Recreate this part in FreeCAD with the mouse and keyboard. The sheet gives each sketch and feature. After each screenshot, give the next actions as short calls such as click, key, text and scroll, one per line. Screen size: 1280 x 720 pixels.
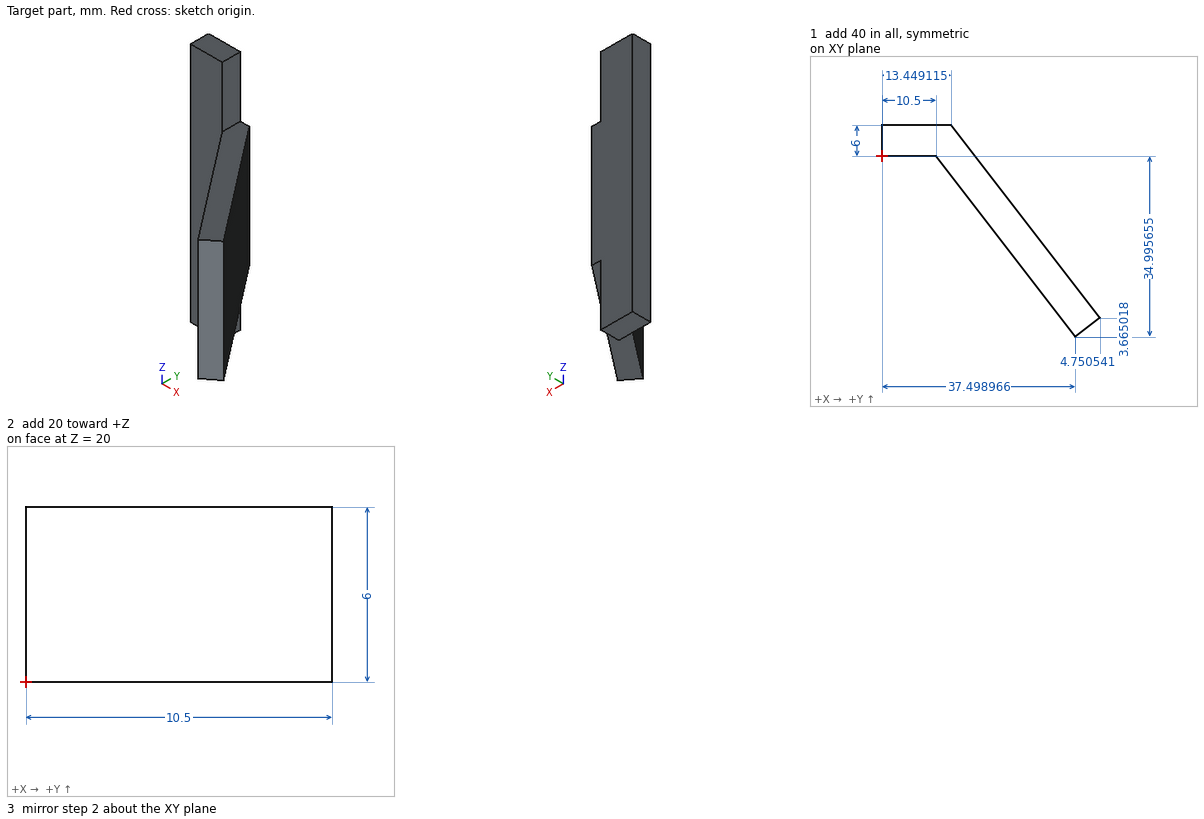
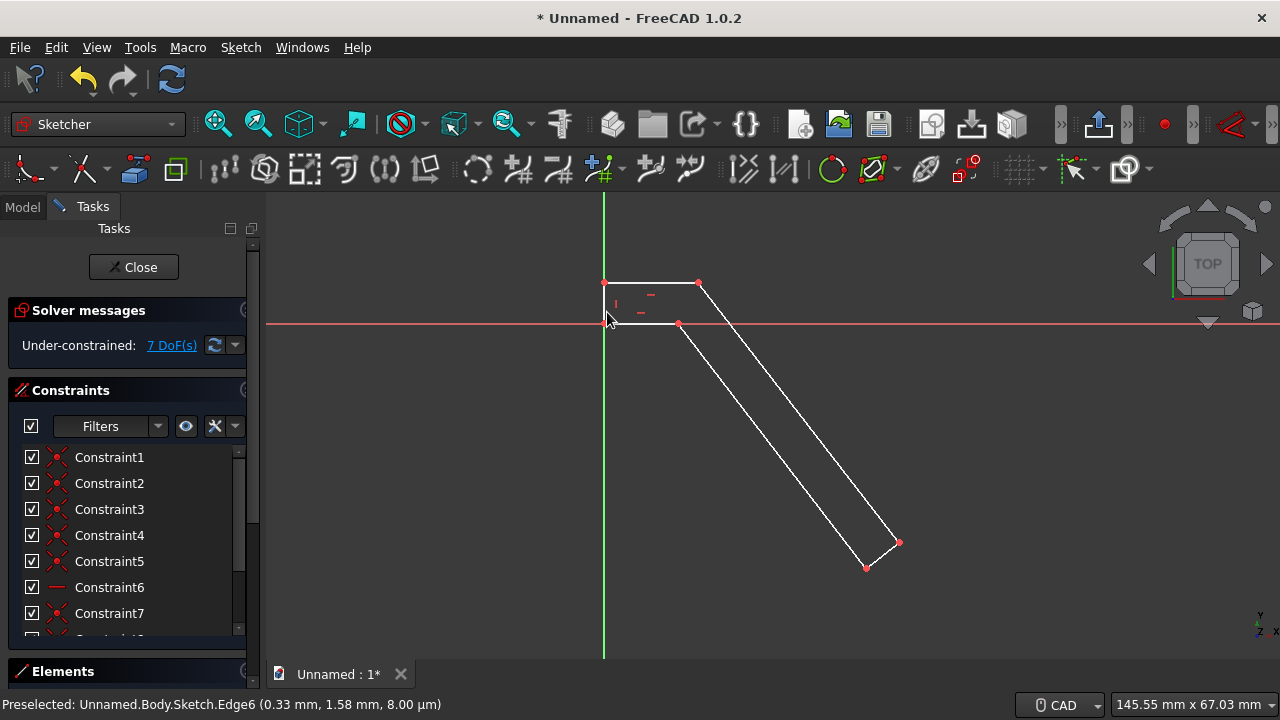
click(1232, 124)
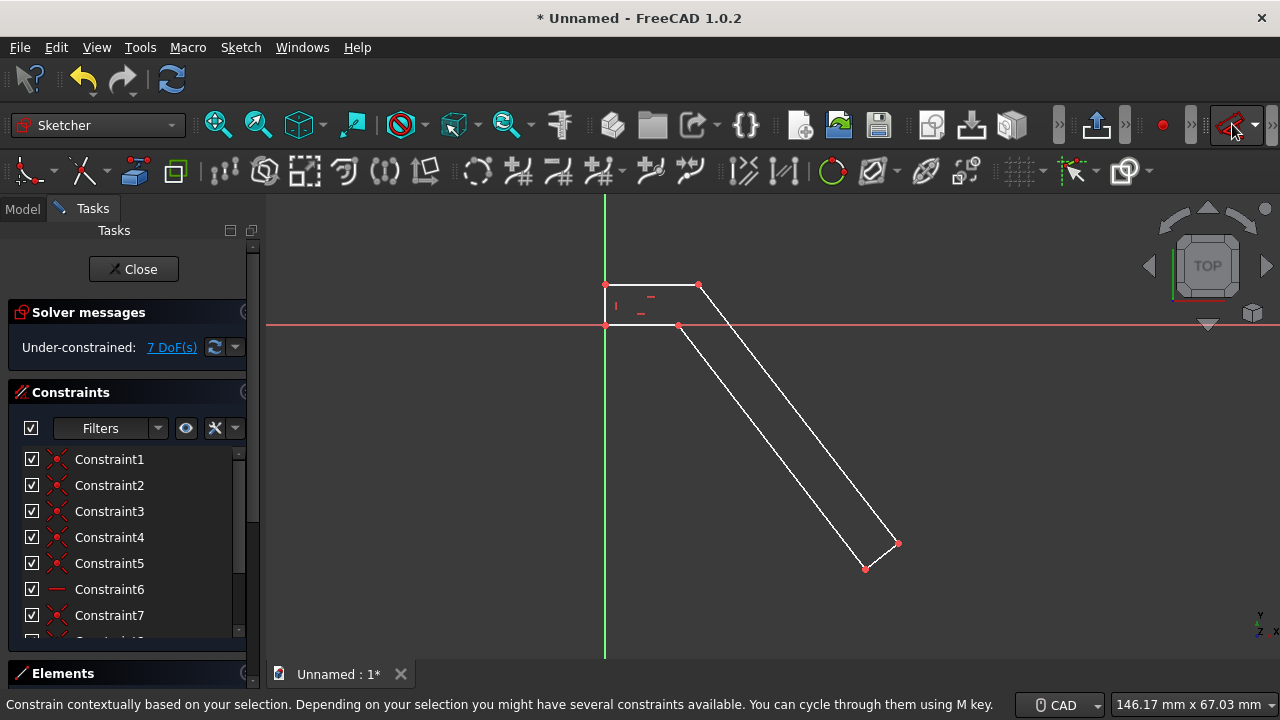
click(605, 297)
click(571, 305)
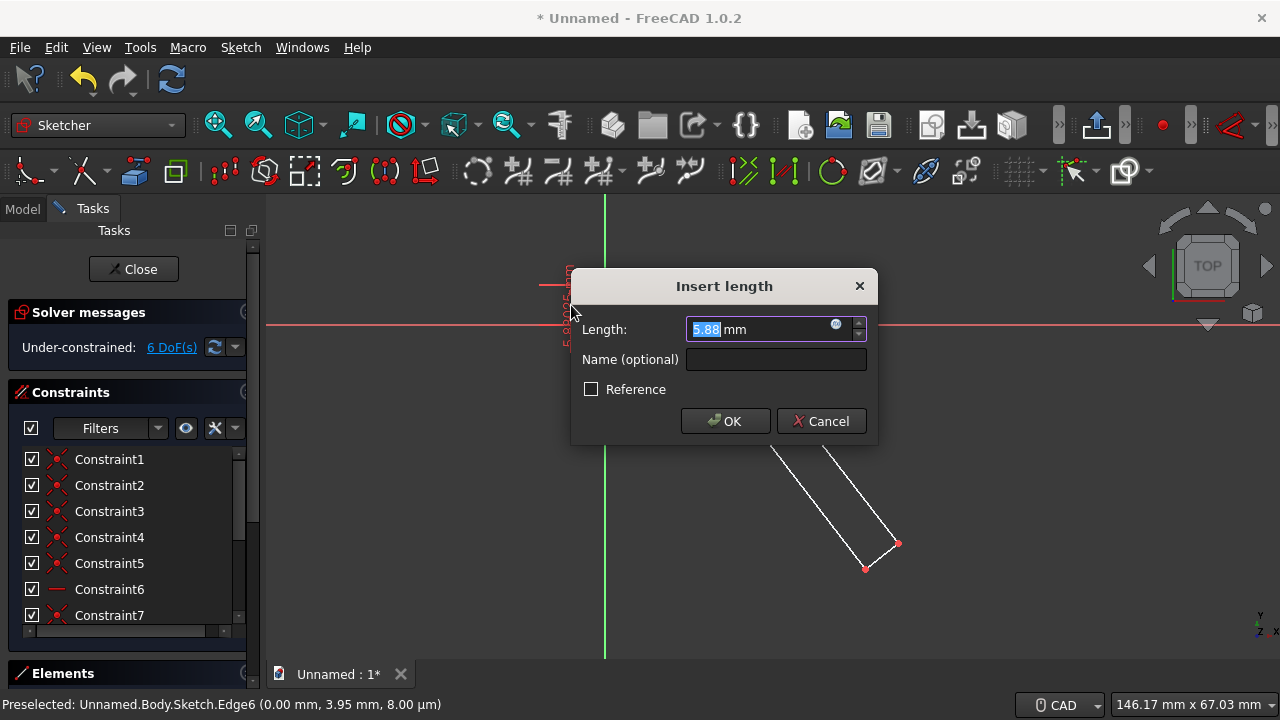
text(6)
key(Return)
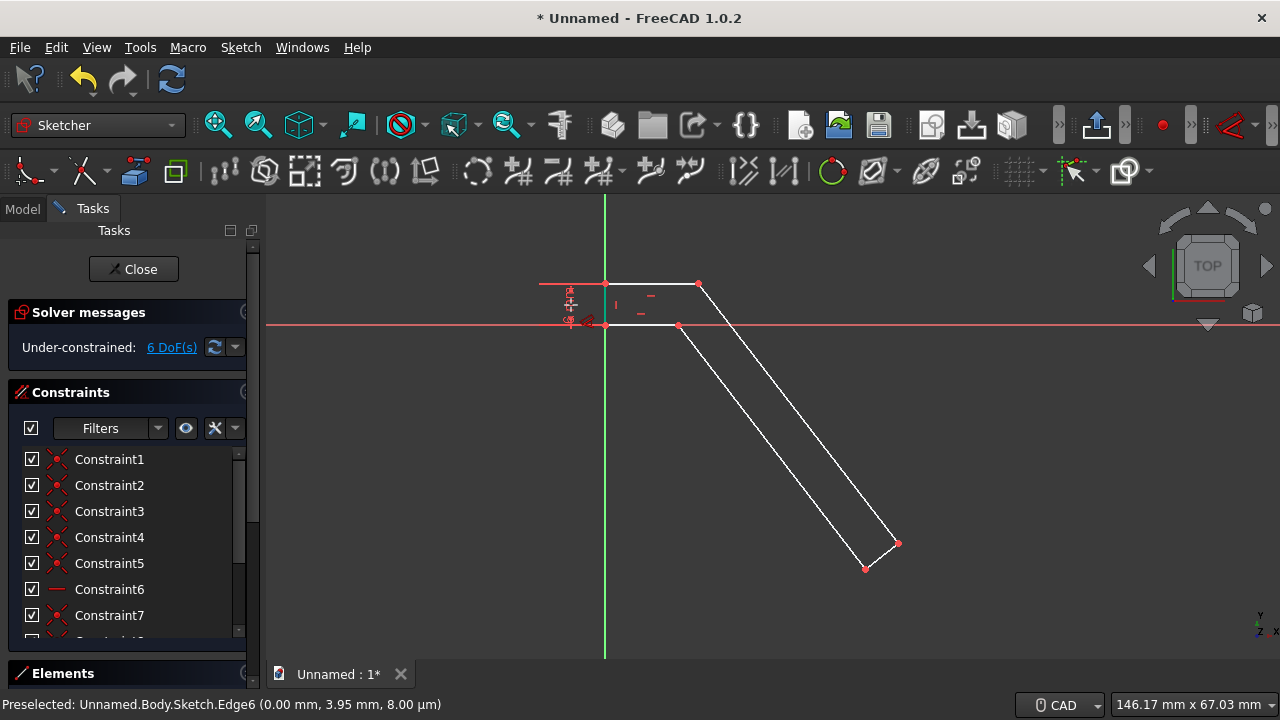
click(627, 325)
click(642, 359)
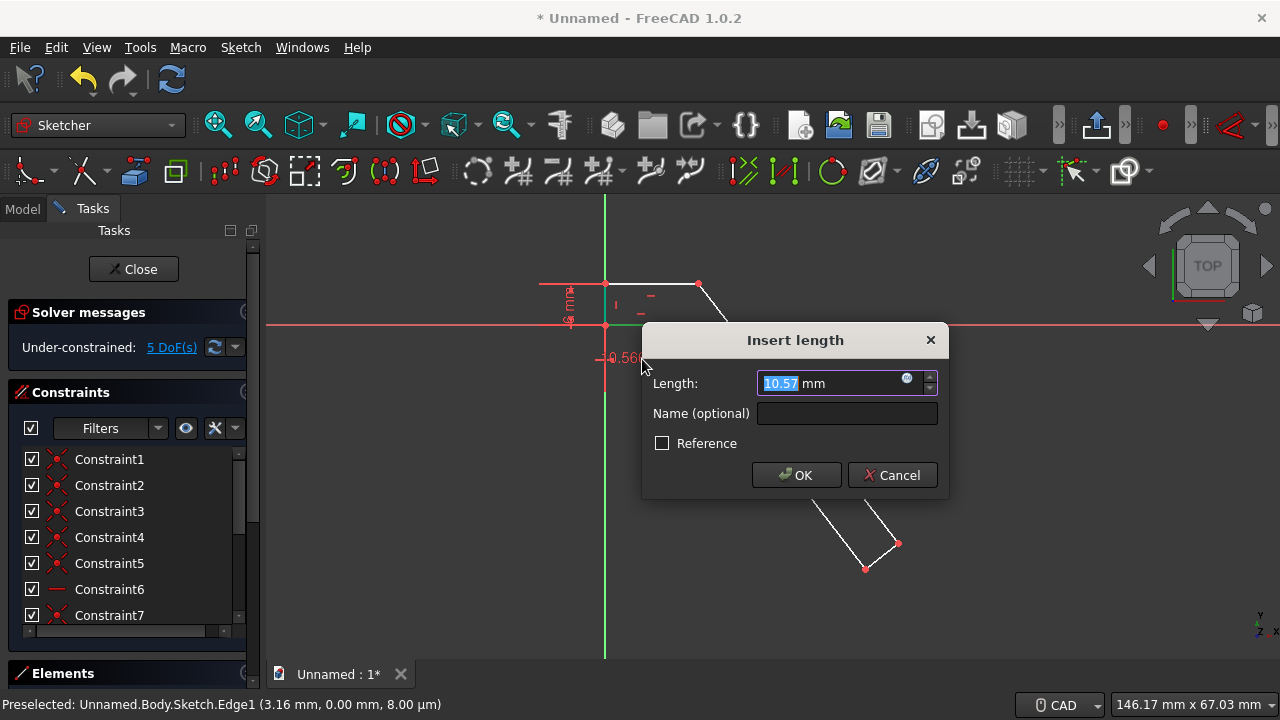
text(10.5)
key(Return)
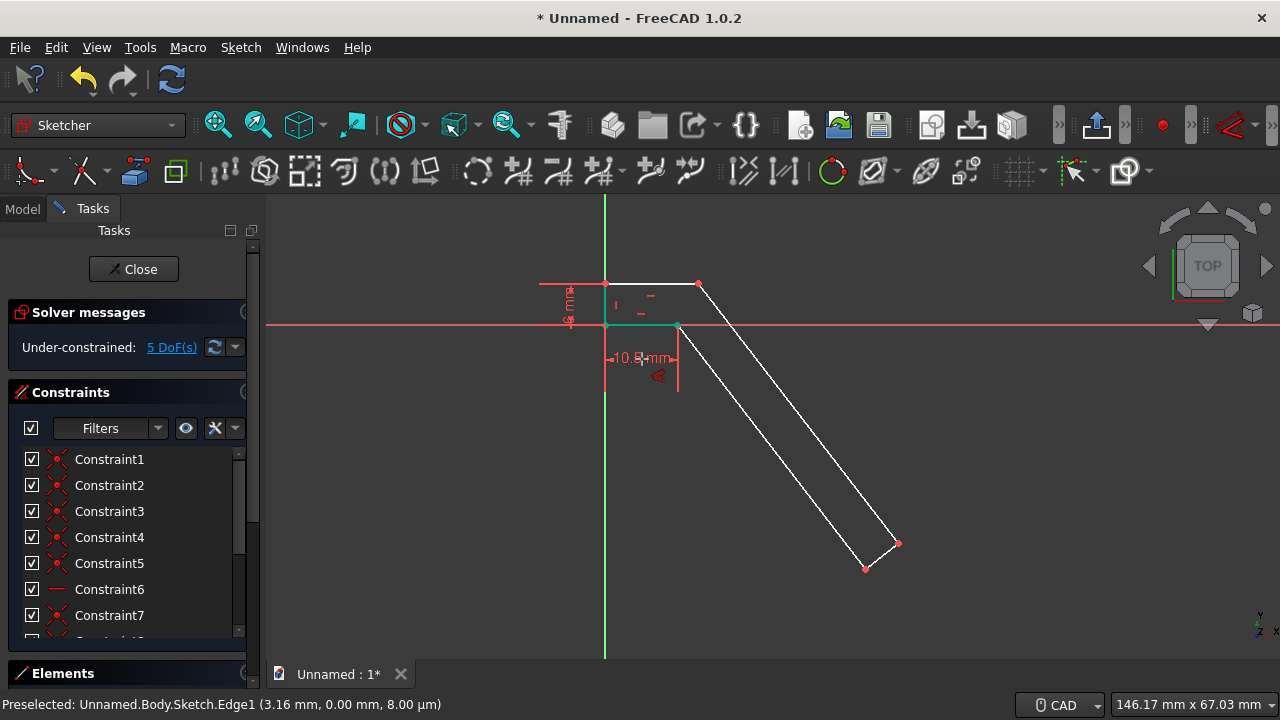
click(670, 284)
click(652, 250)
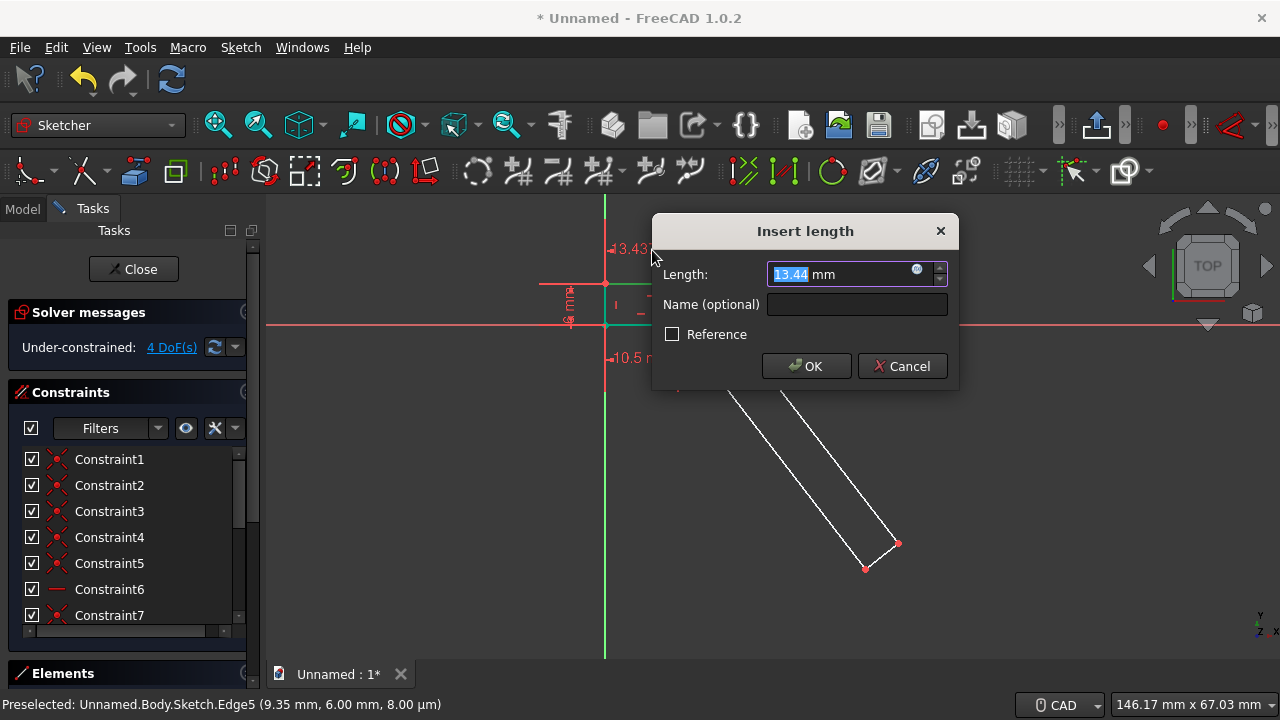
text(13.449115)
key(Return)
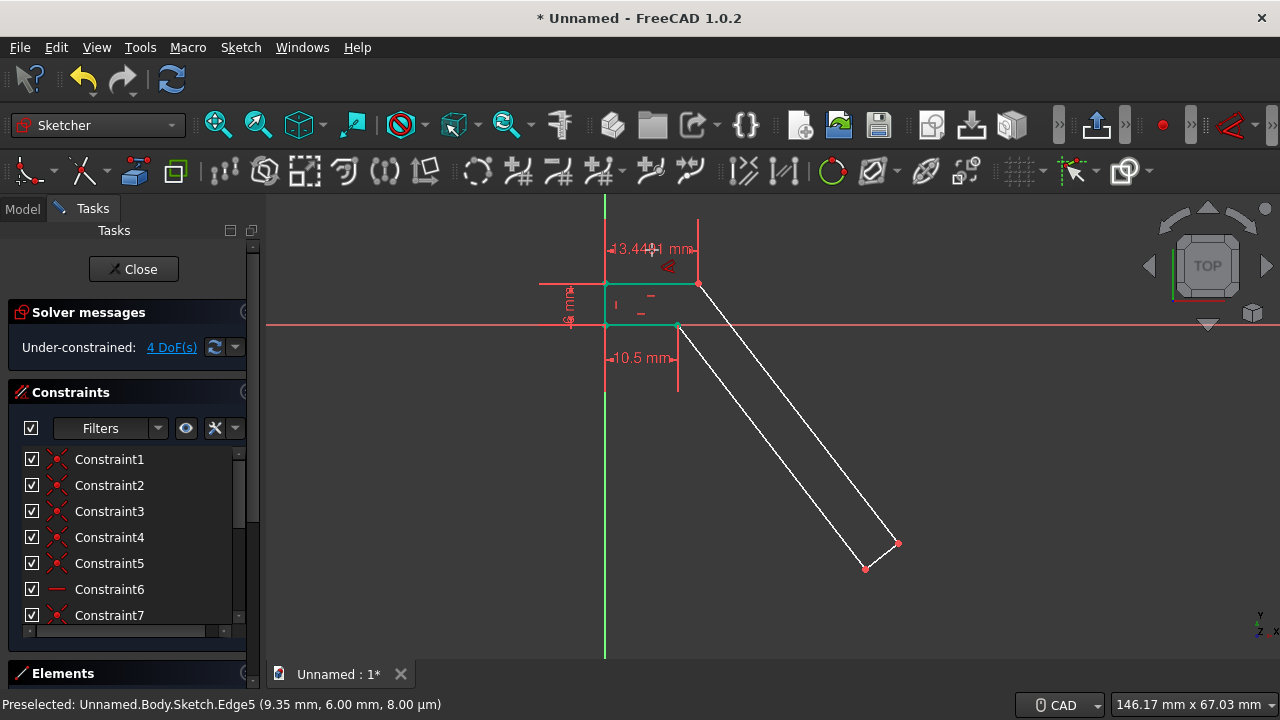
click(875, 562)
click(882, 603)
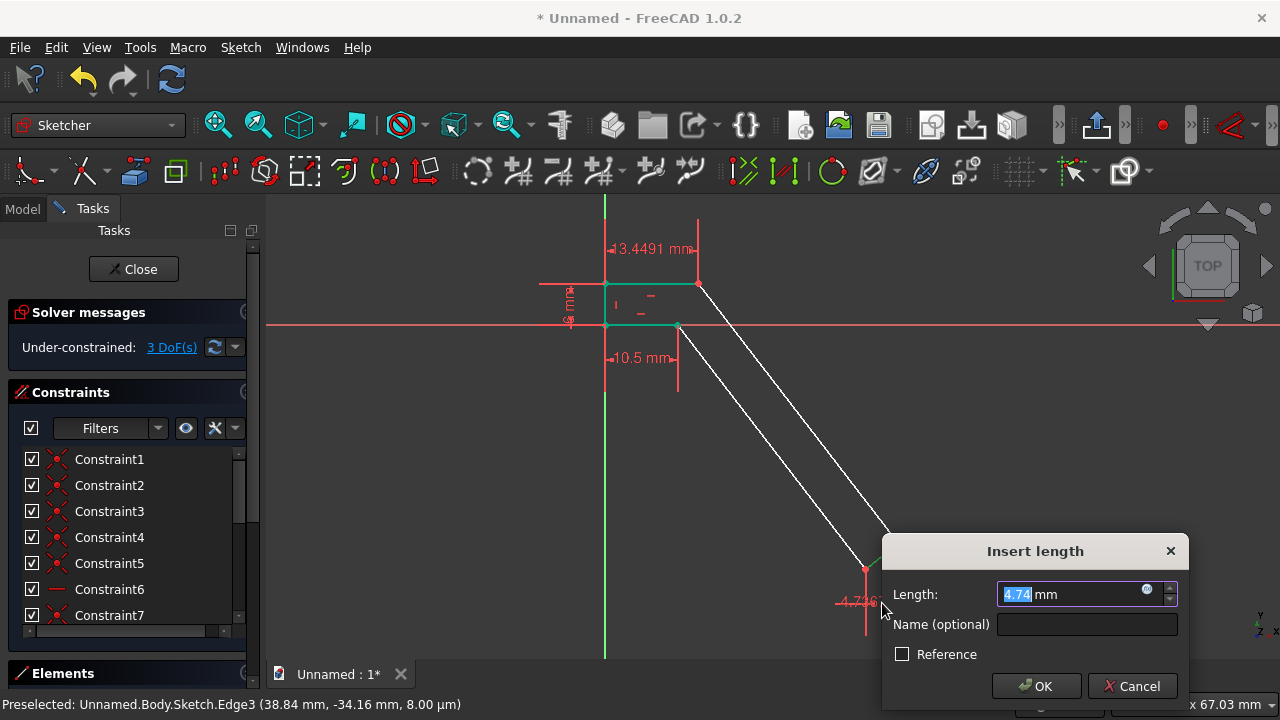
text(4.750541)
key(Return)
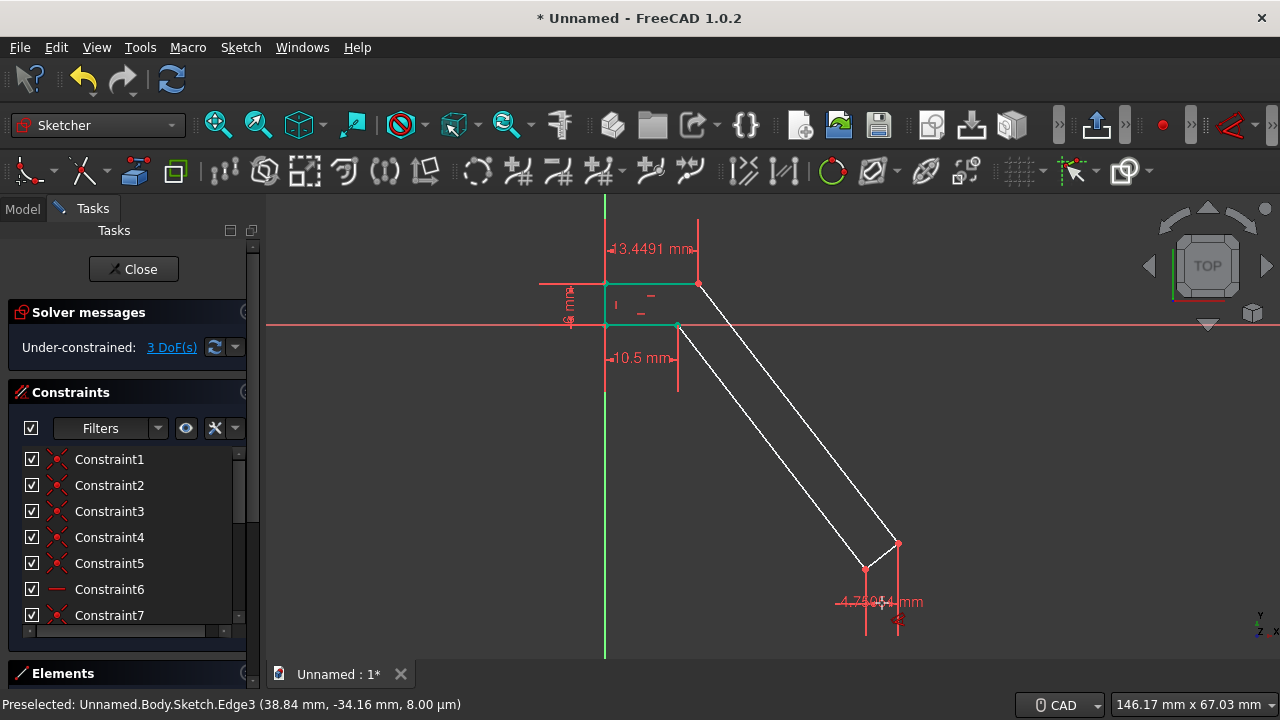
scroll(875, 562, up, 3)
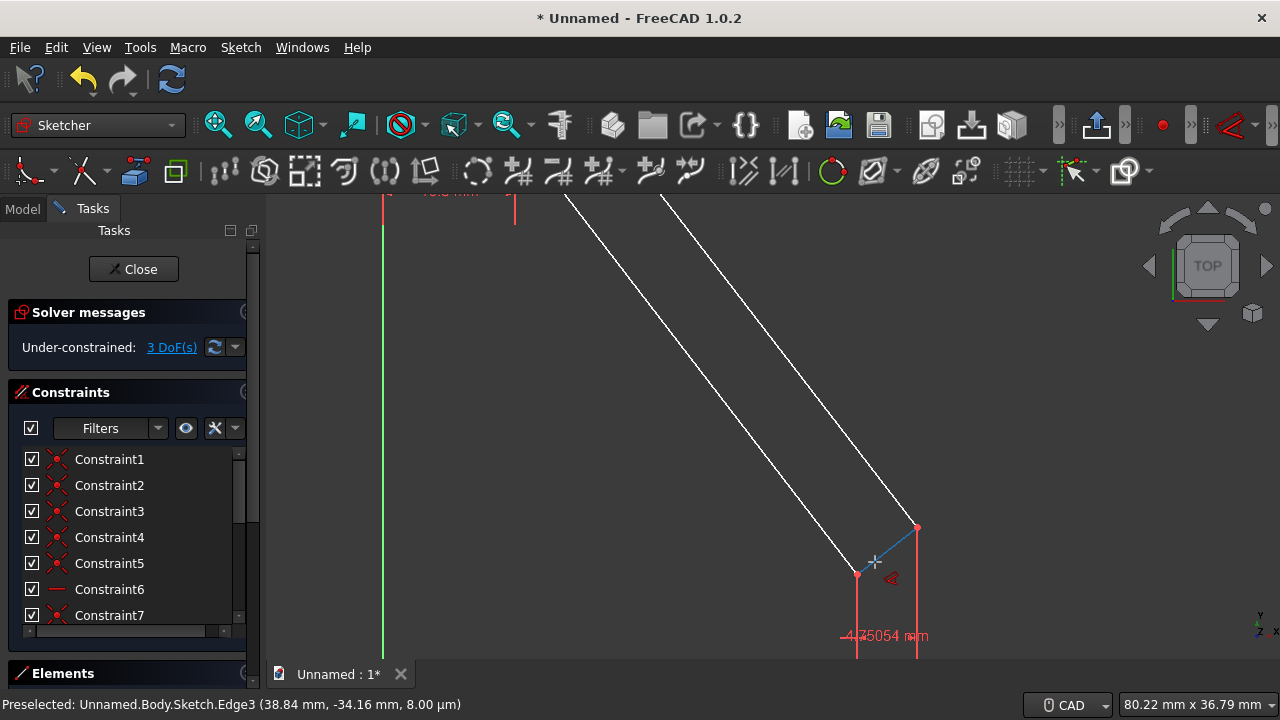
click(875, 561)
click(951, 551)